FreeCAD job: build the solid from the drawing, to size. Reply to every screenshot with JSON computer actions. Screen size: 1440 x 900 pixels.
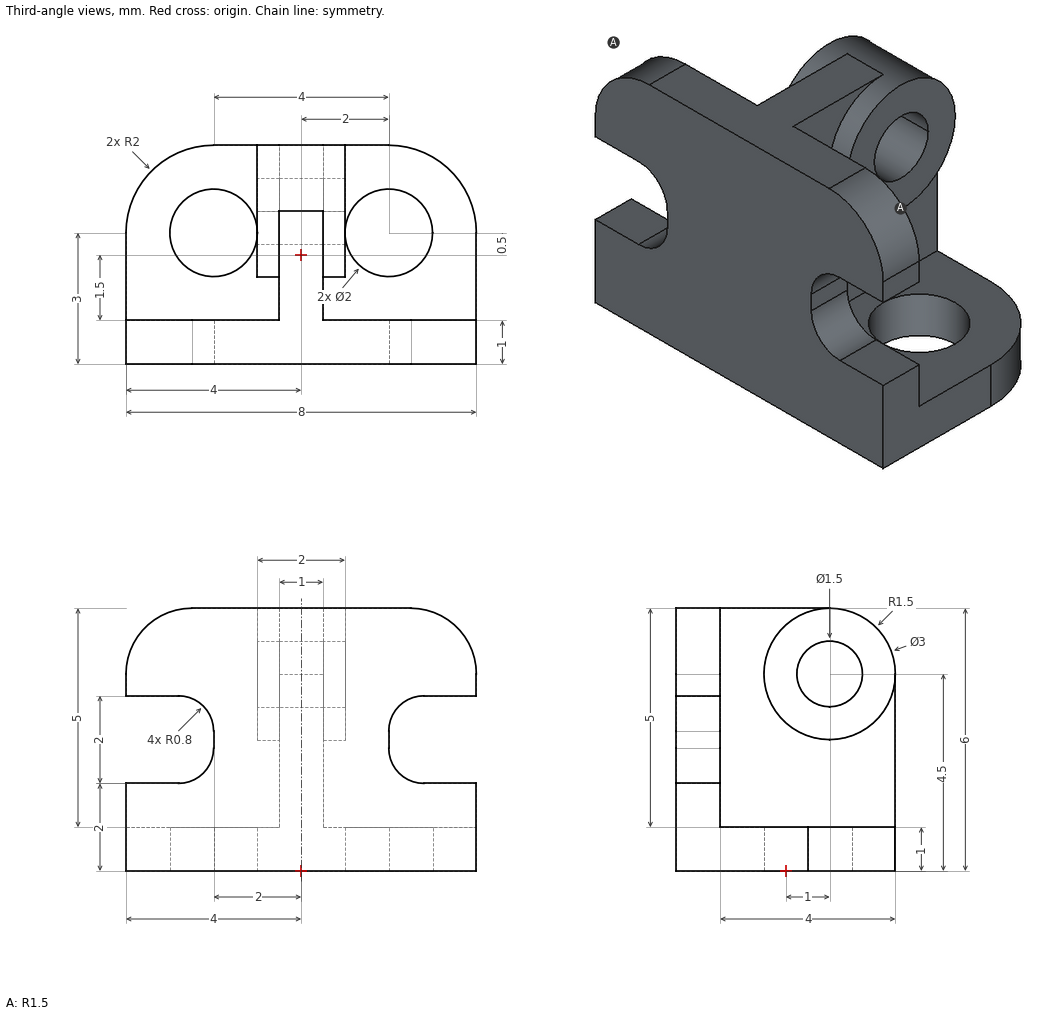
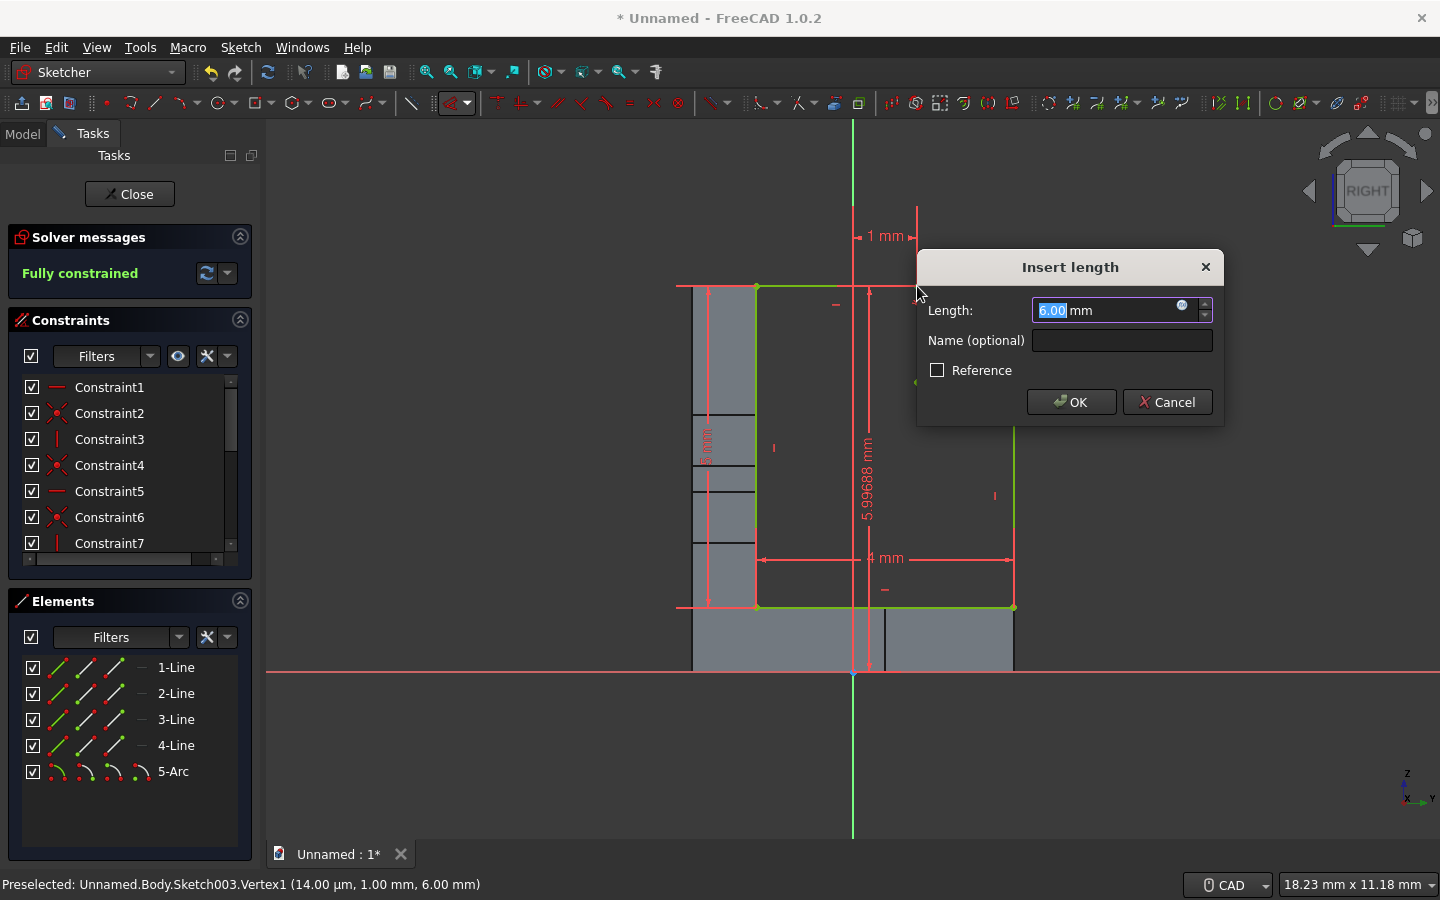
{"action": "type", "text": "6"}
{"action": "key", "text": "Return"}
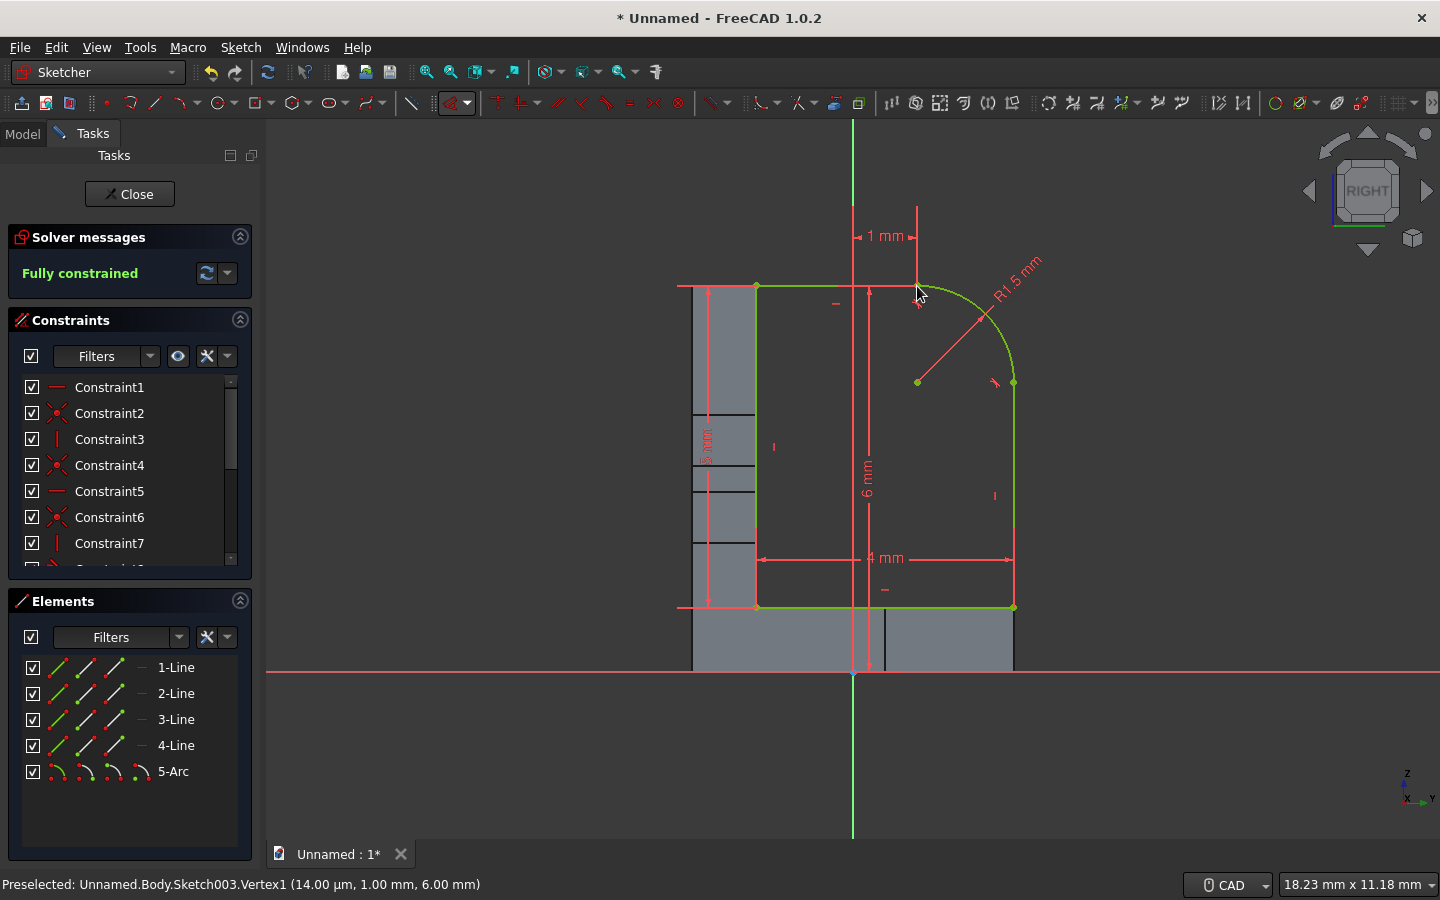
{"action": "left_click", "coordinate": [130, 194]}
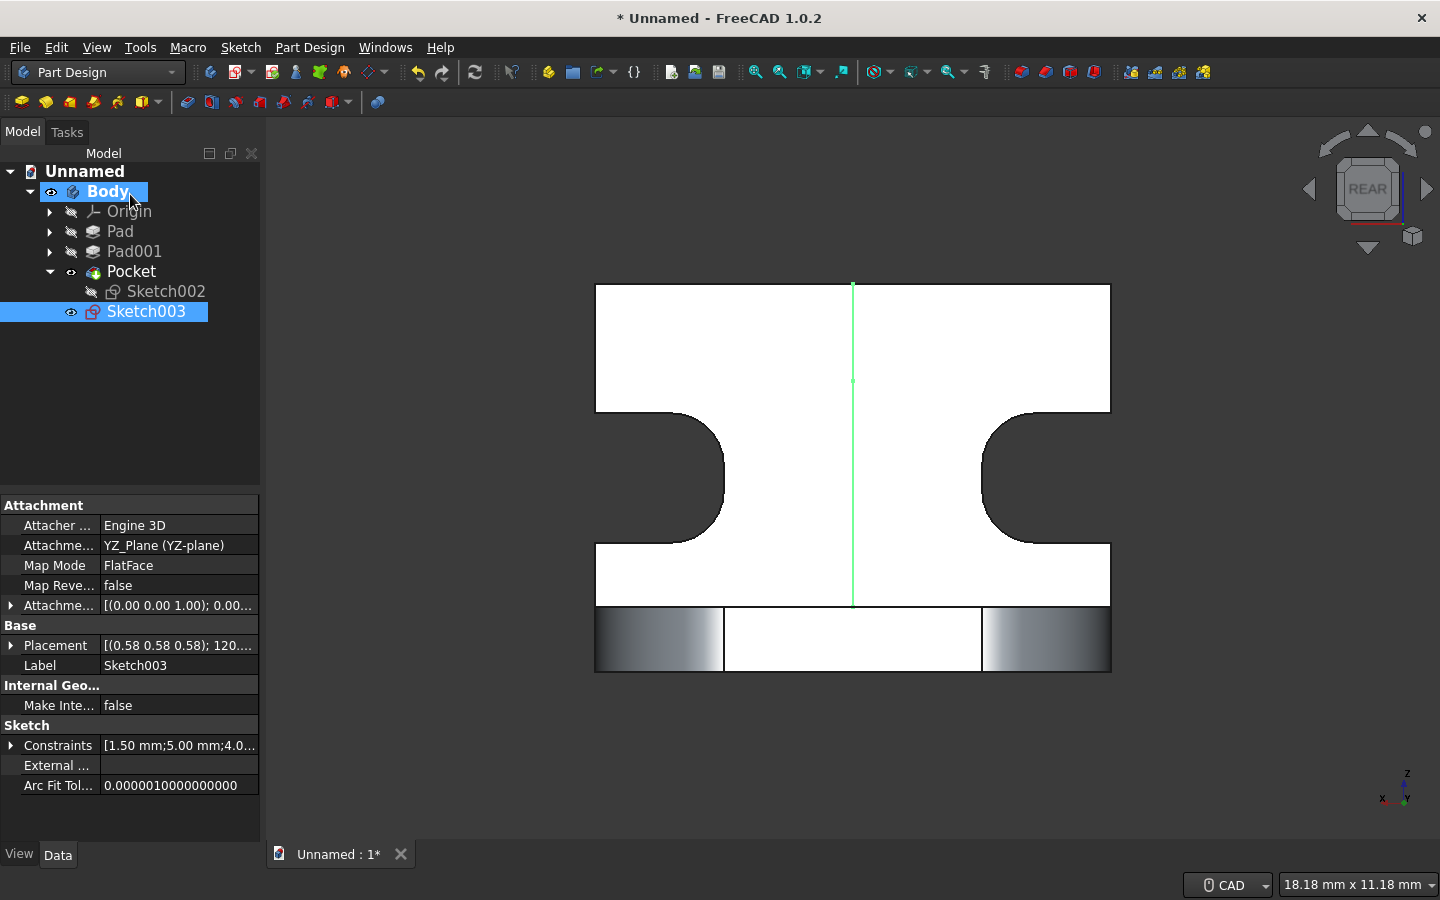
{"action": "left_click", "coordinate": [22, 102]}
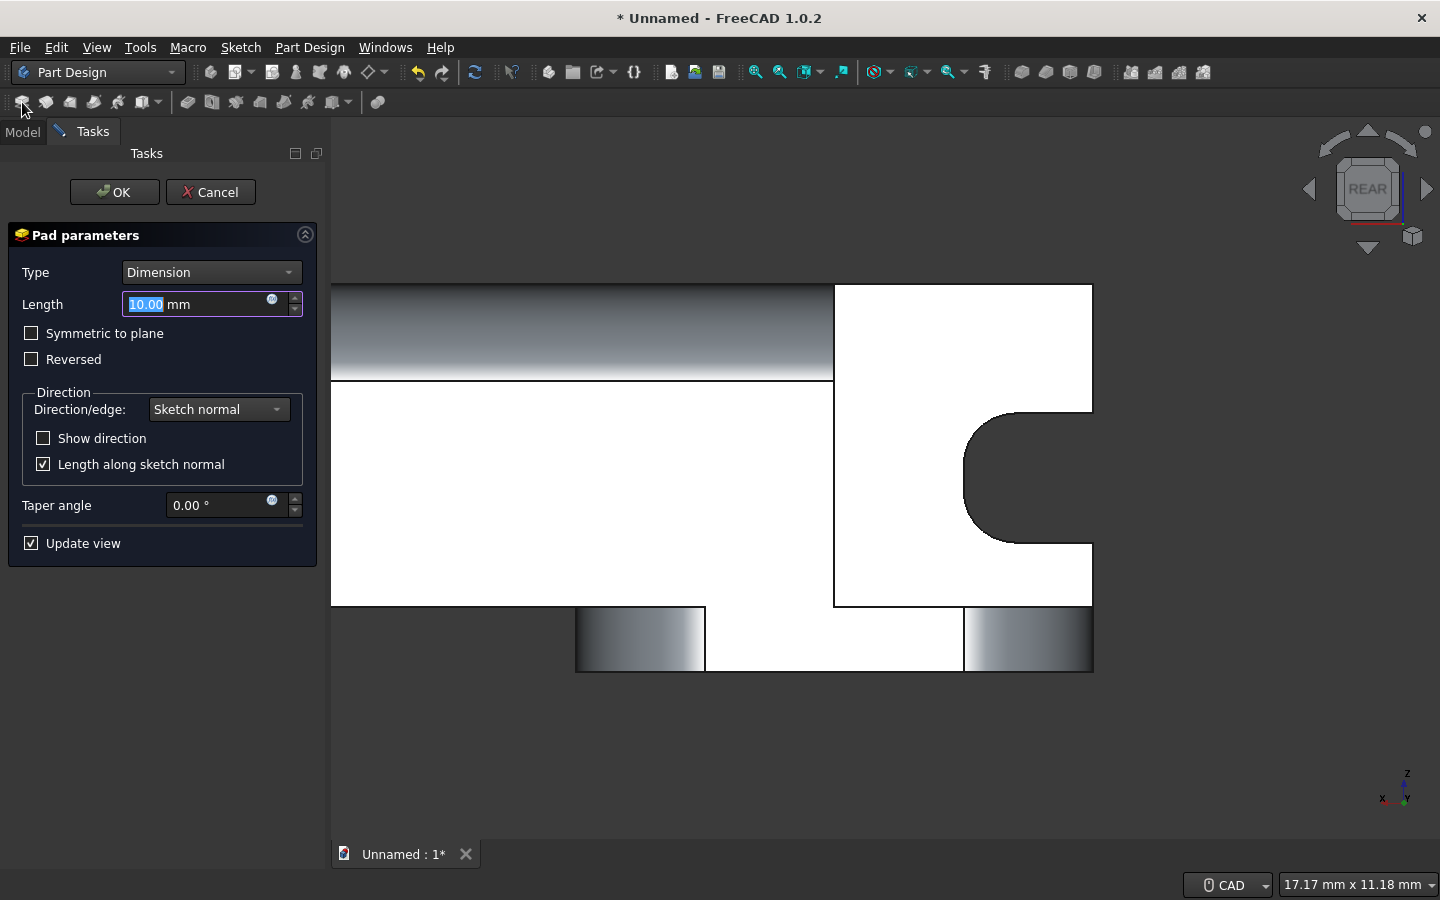
{"action": "type", "text": "1"}
{"action": "key", "text": "Tab"}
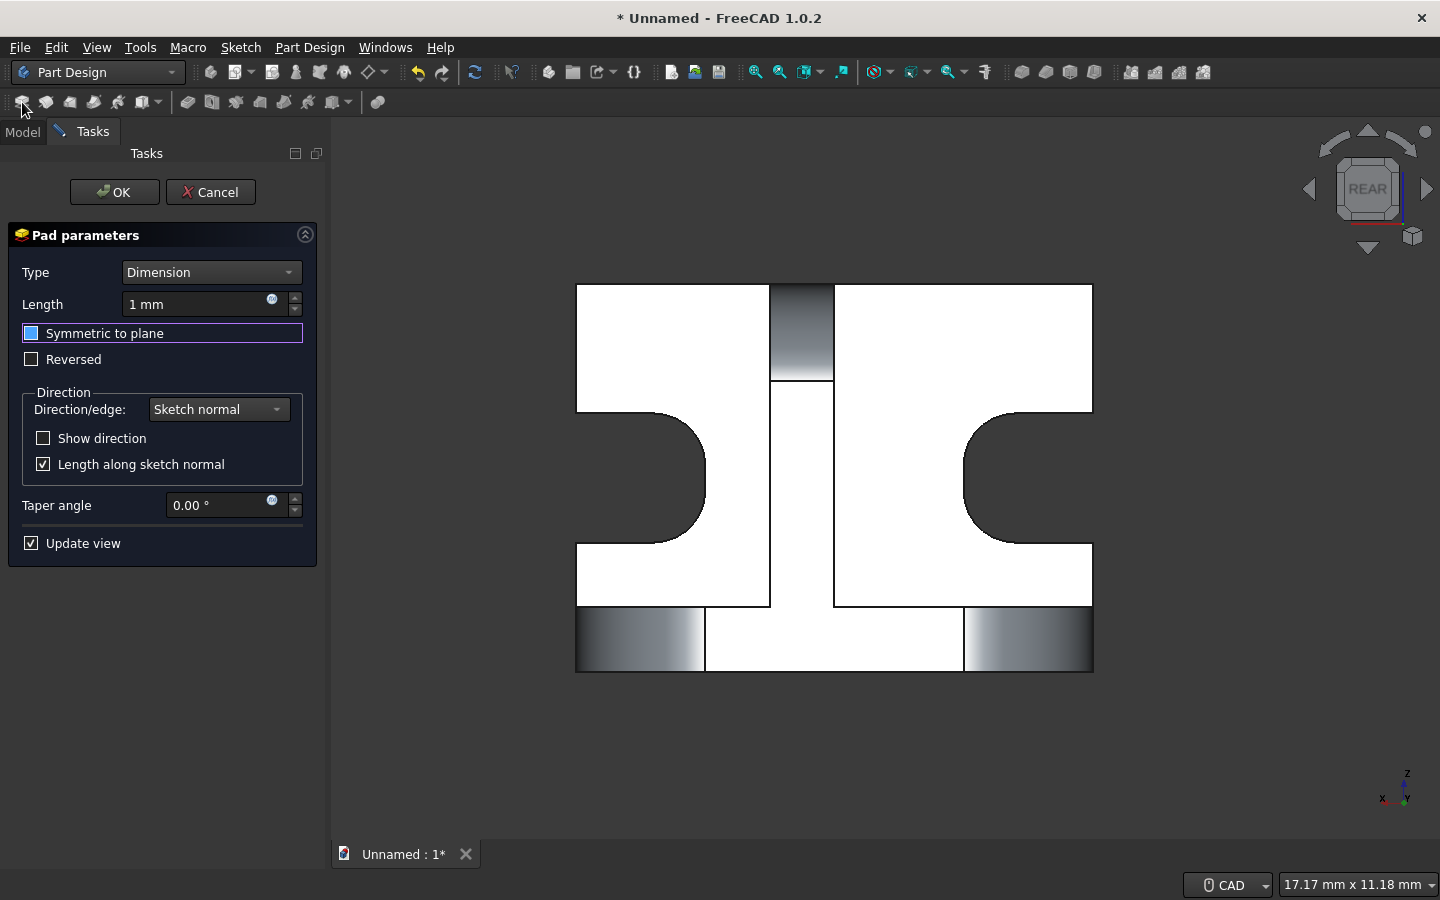
{"action": "left_click", "coordinate": [30, 333]}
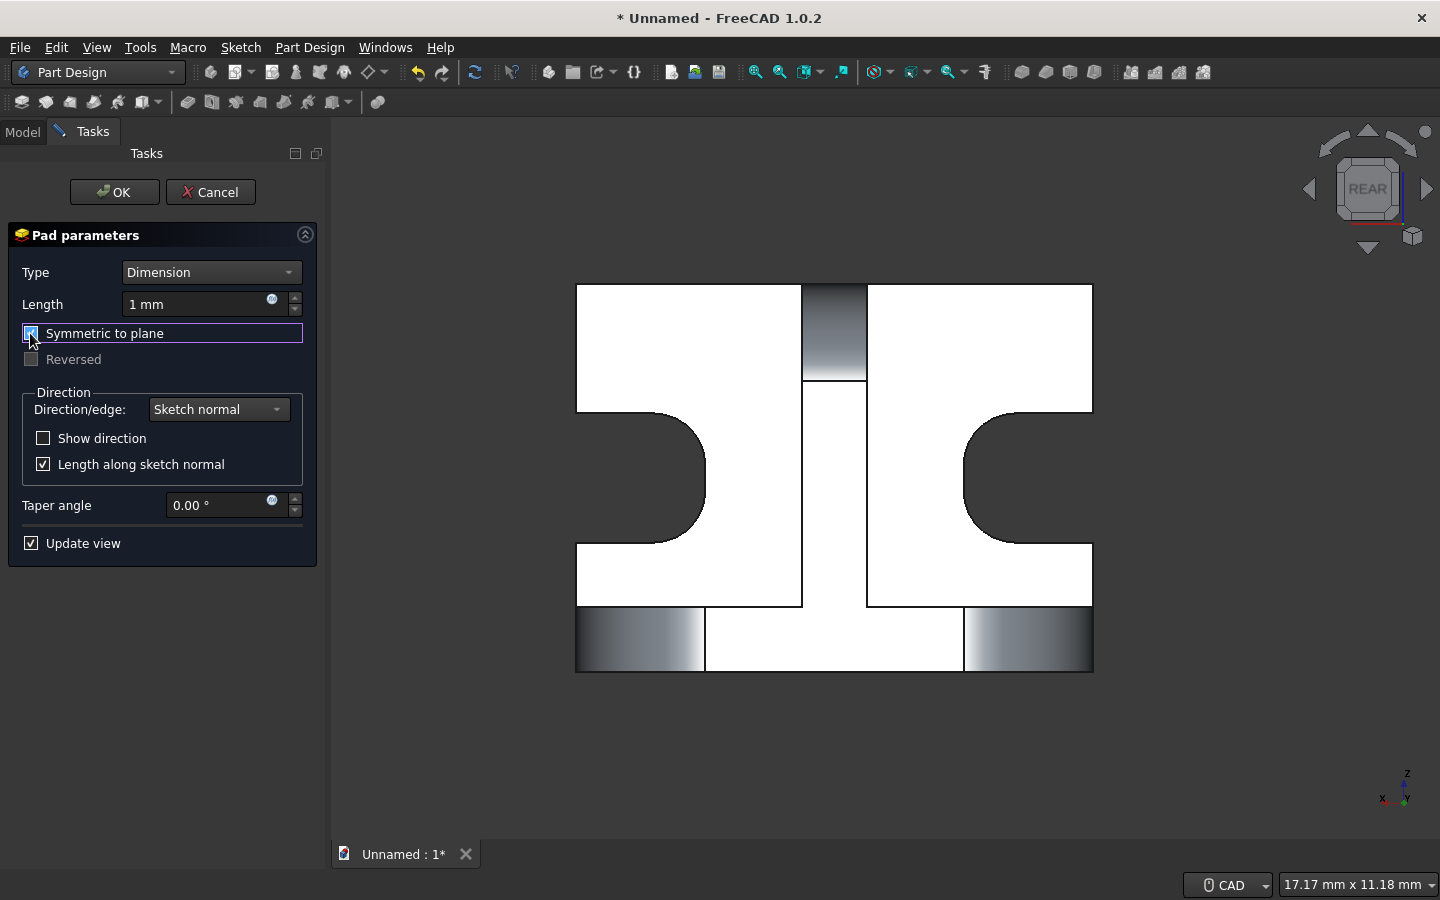
{"action": "left_click", "coordinate": [115, 192]}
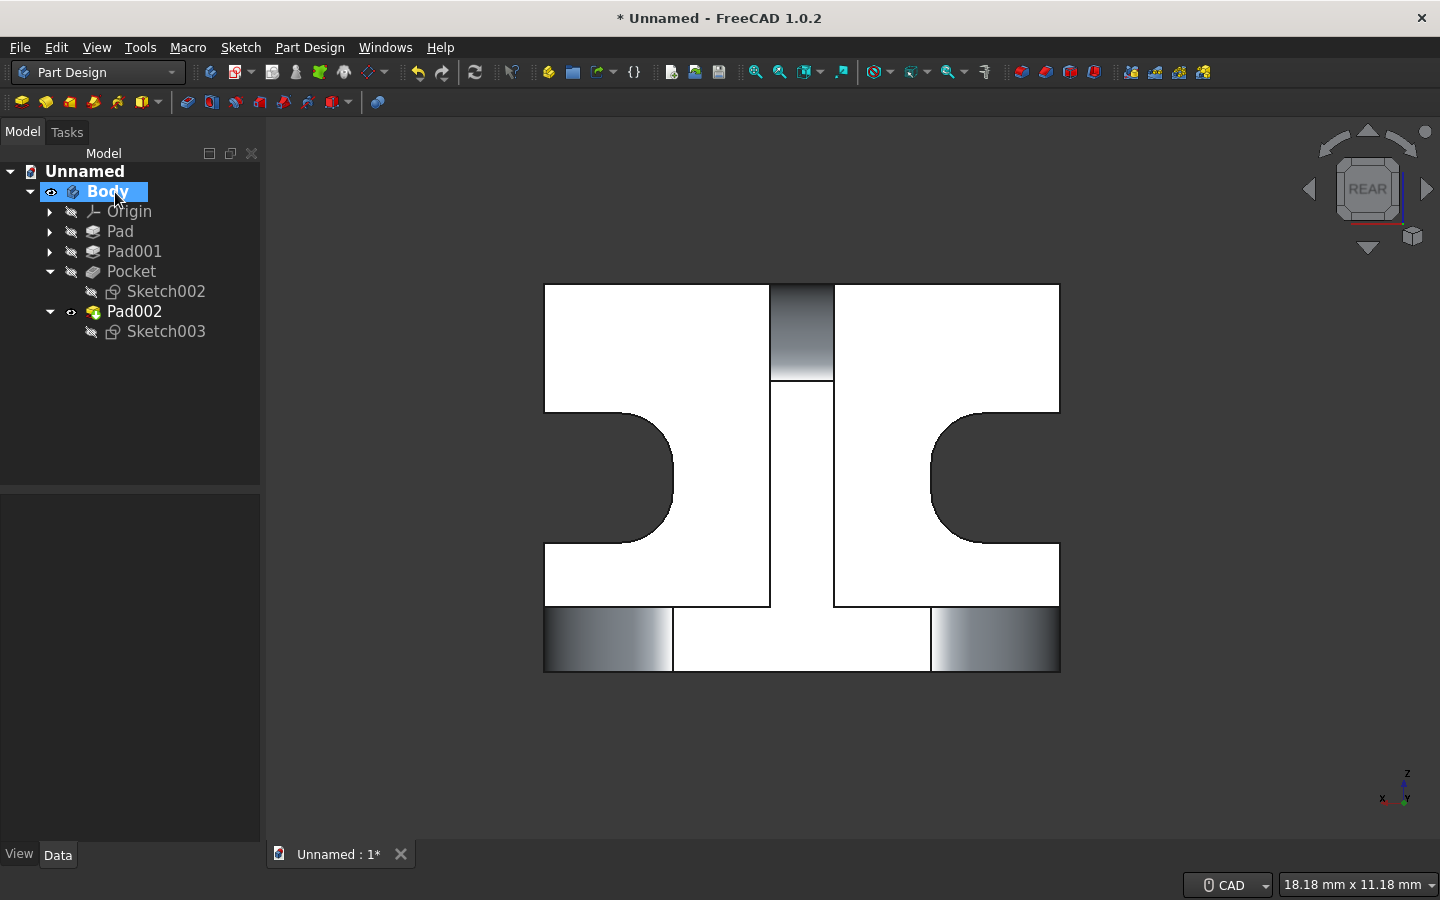
{"action": "left_click", "coordinate": [236, 72]}